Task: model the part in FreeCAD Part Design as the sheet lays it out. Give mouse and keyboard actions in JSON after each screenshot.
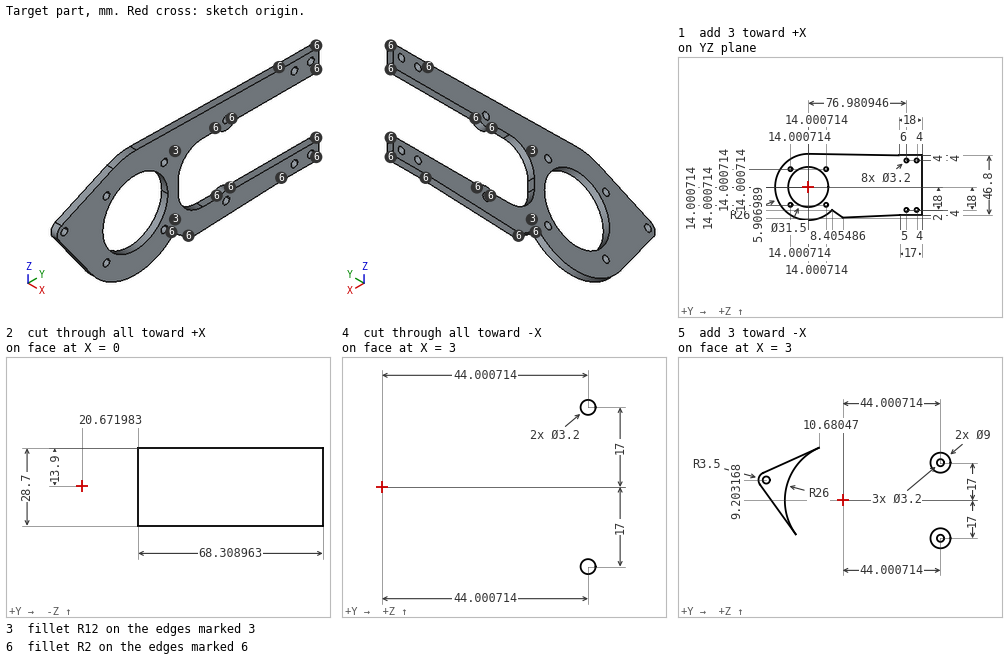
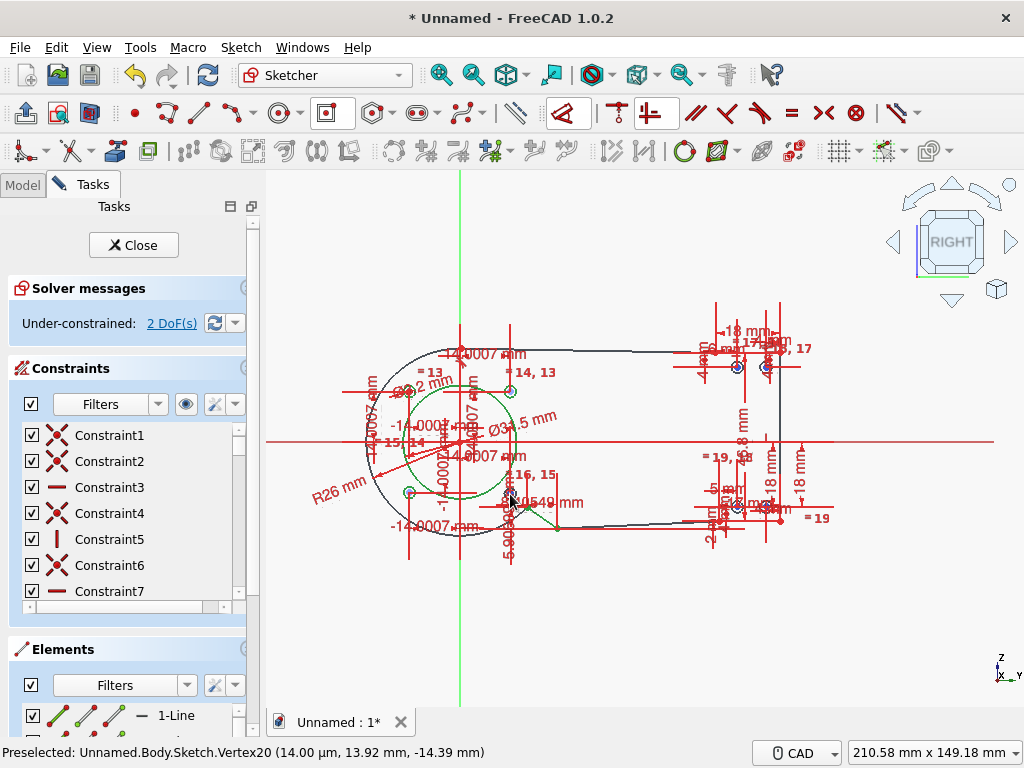
{"action": "left_click", "coordinate": [510, 494]}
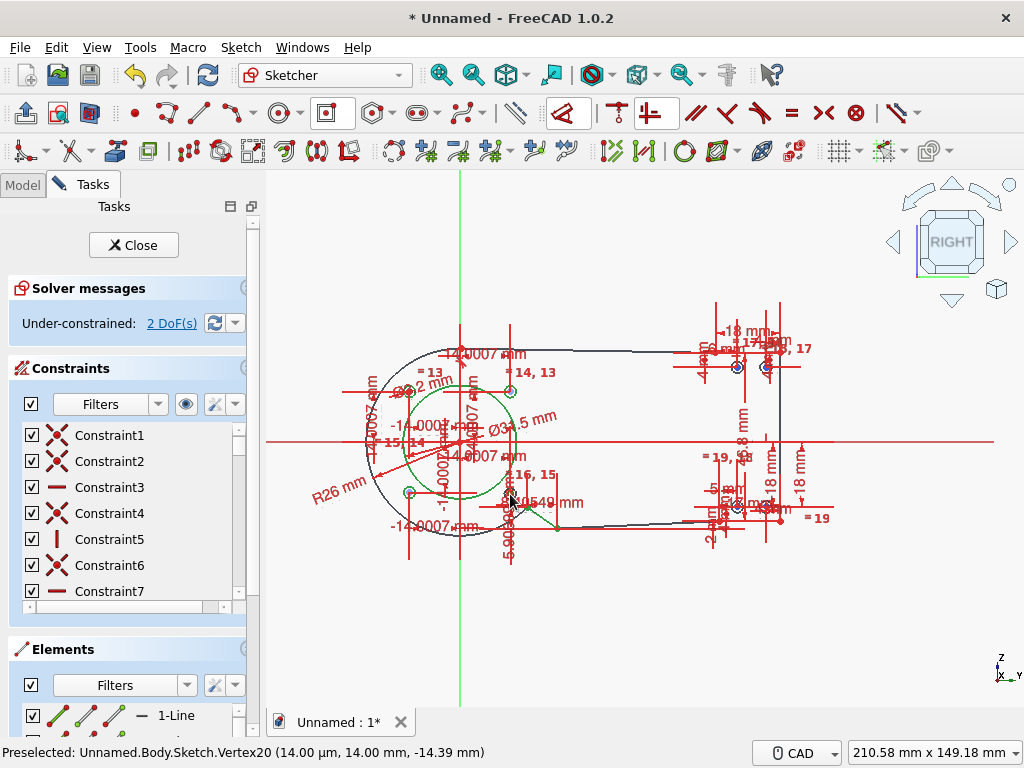
{"action": "key", "text": "i"}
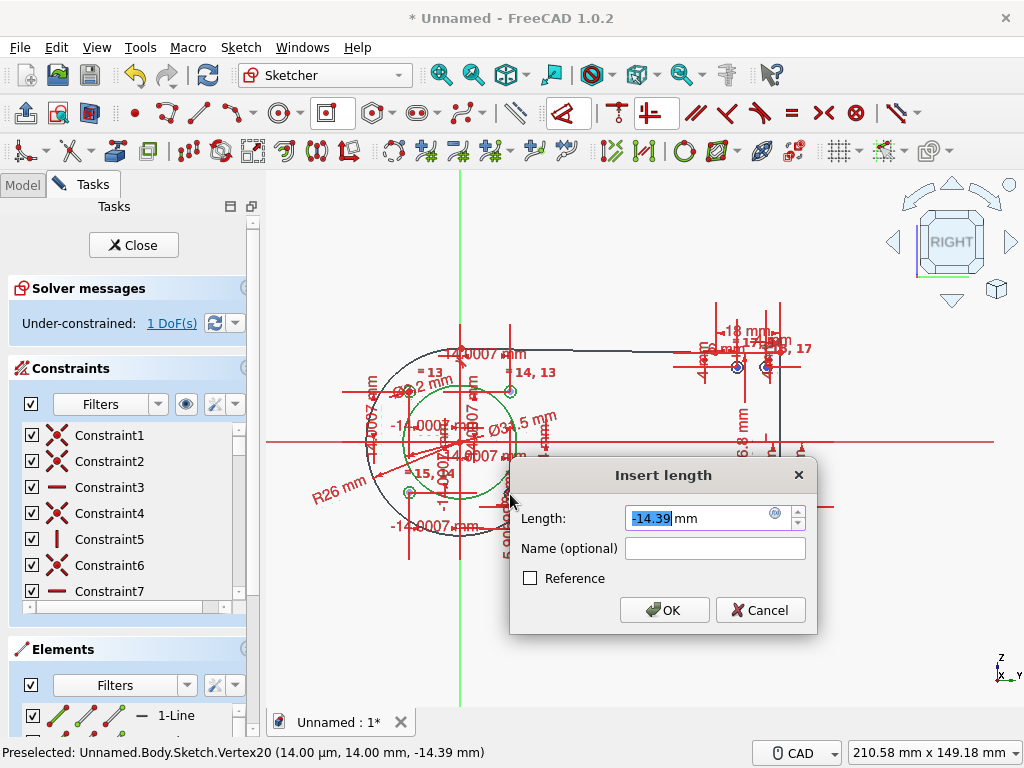
{"action": "type", "text": "-14.000714"}
{"action": "key", "text": "Return"}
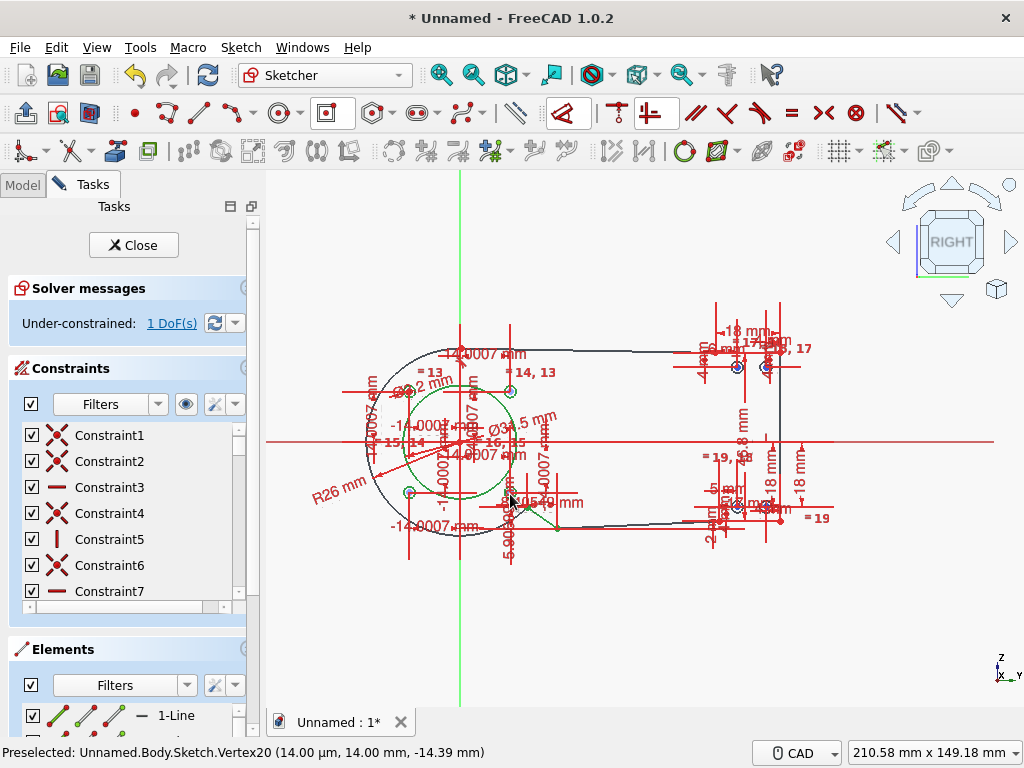
{"action": "left_click", "coordinate": [737, 367]}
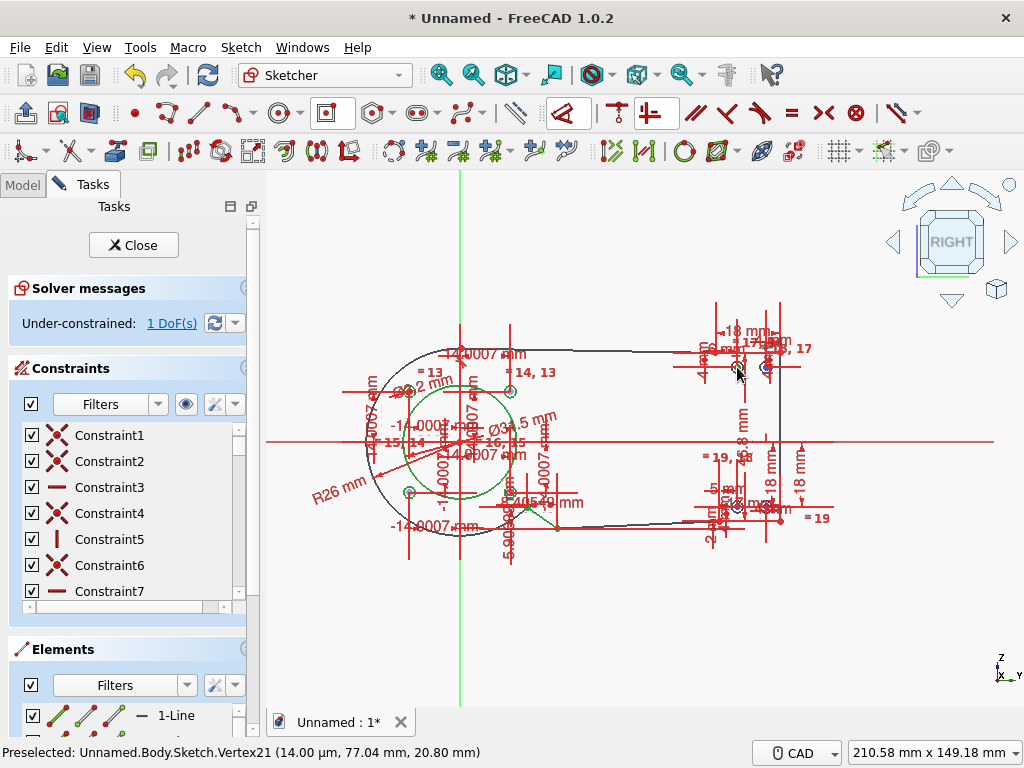
{"action": "key", "text": "l"}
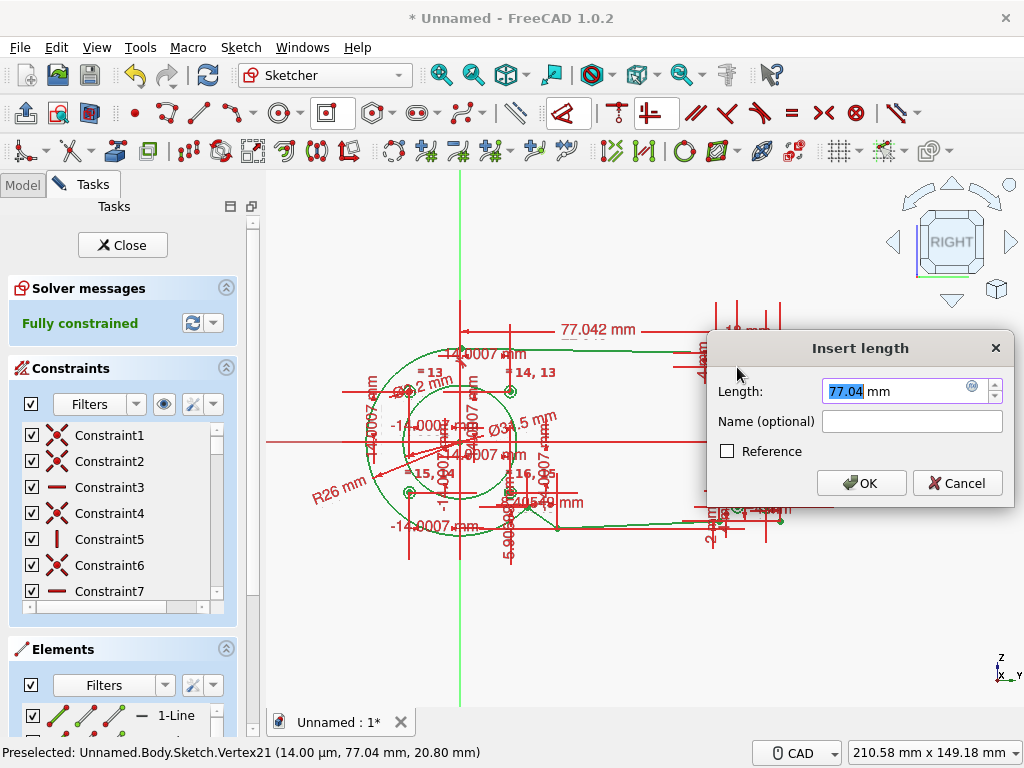
{"action": "type", "text": "76.980946"}
{"action": "key", "text": "Return"}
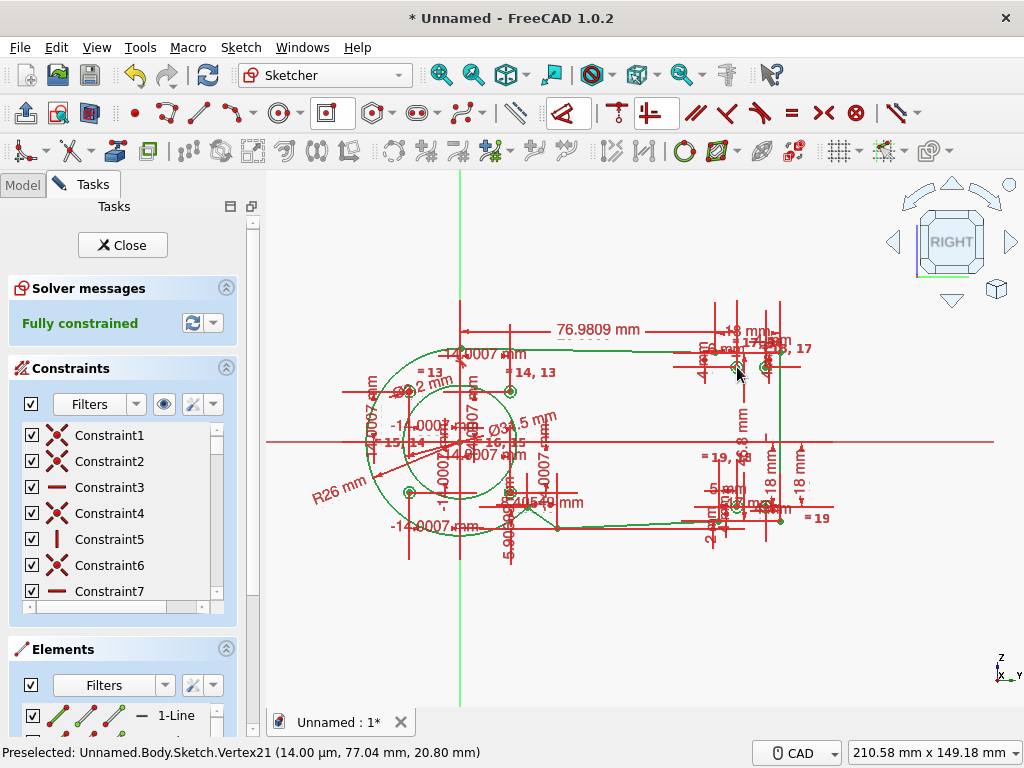
{"action": "left_click", "coordinate": [123, 245]}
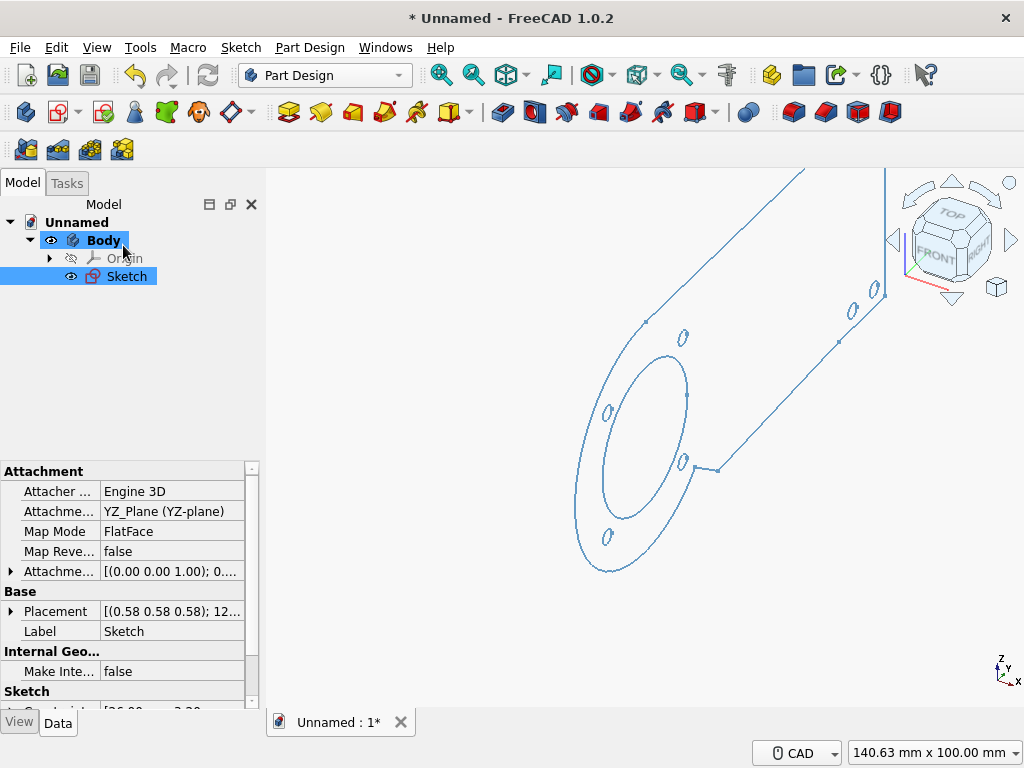
{"action": "left_click", "coordinate": [290, 112]}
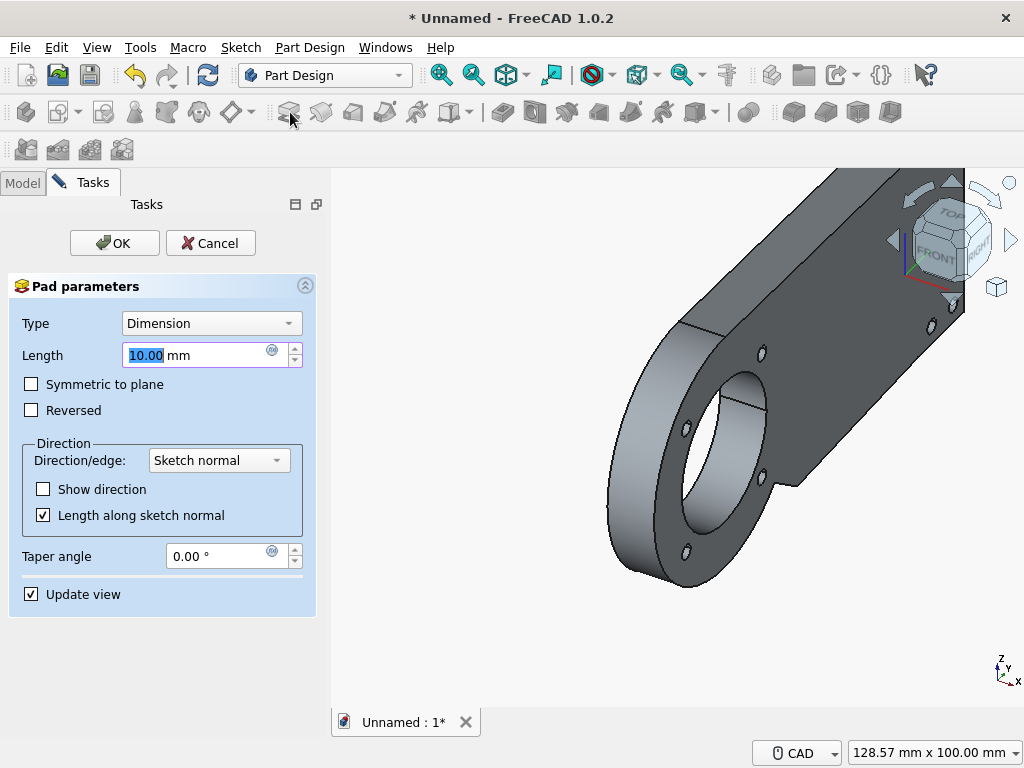
{"action": "type", "text": "3"}
{"action": "key", "text": "Tab"}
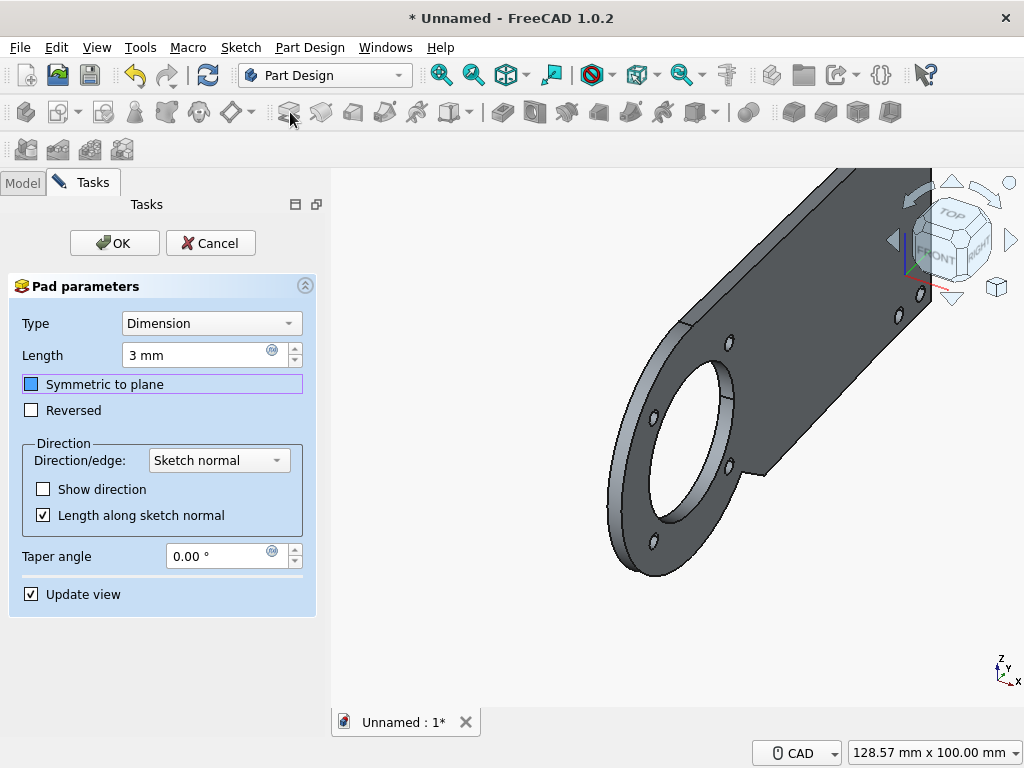
{"action": "left_click", "coordinate": [115, 243]}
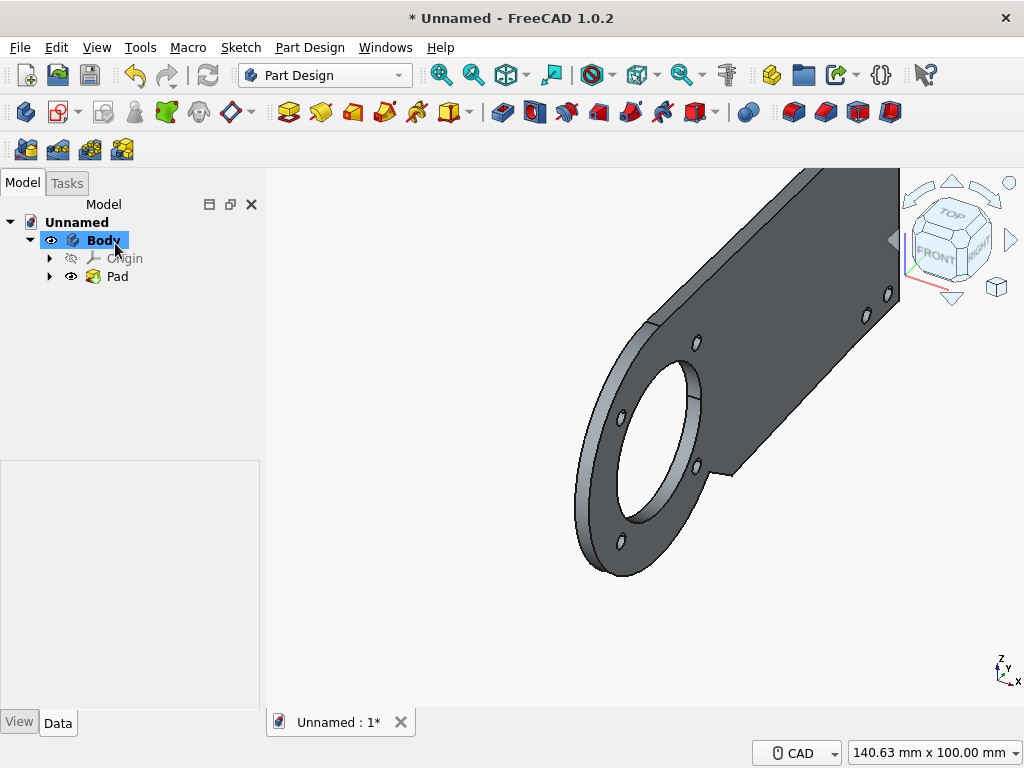
{"action": "left_click", "coordinate": [442, 76]}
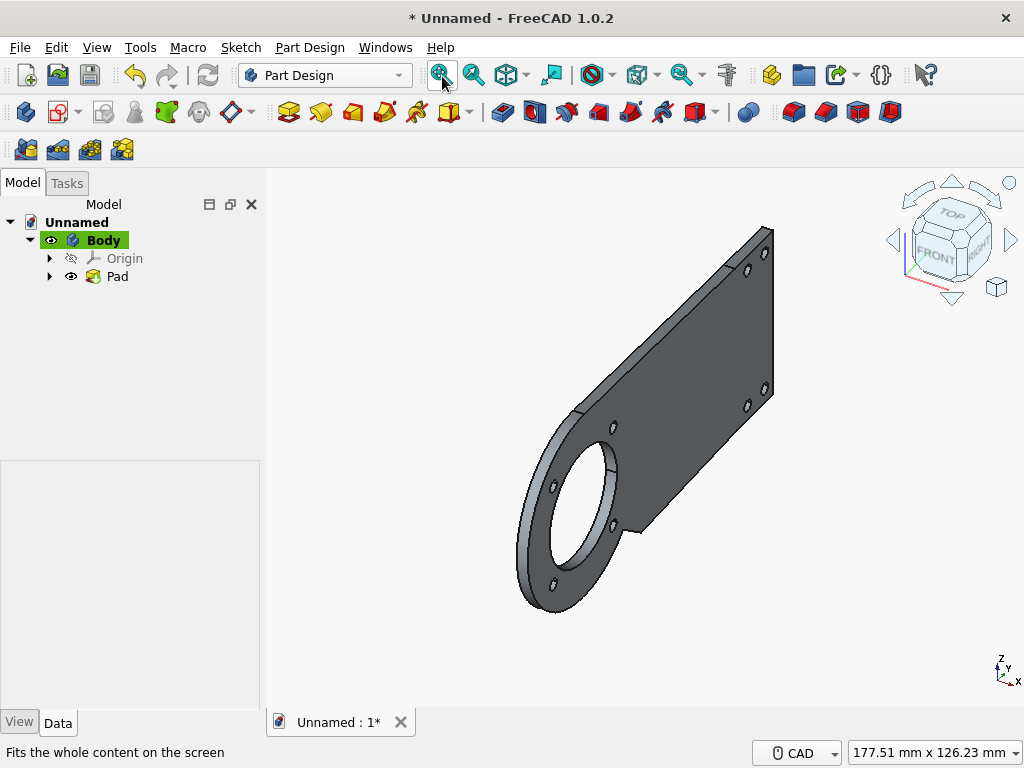
{"action": "key", "text": "6"}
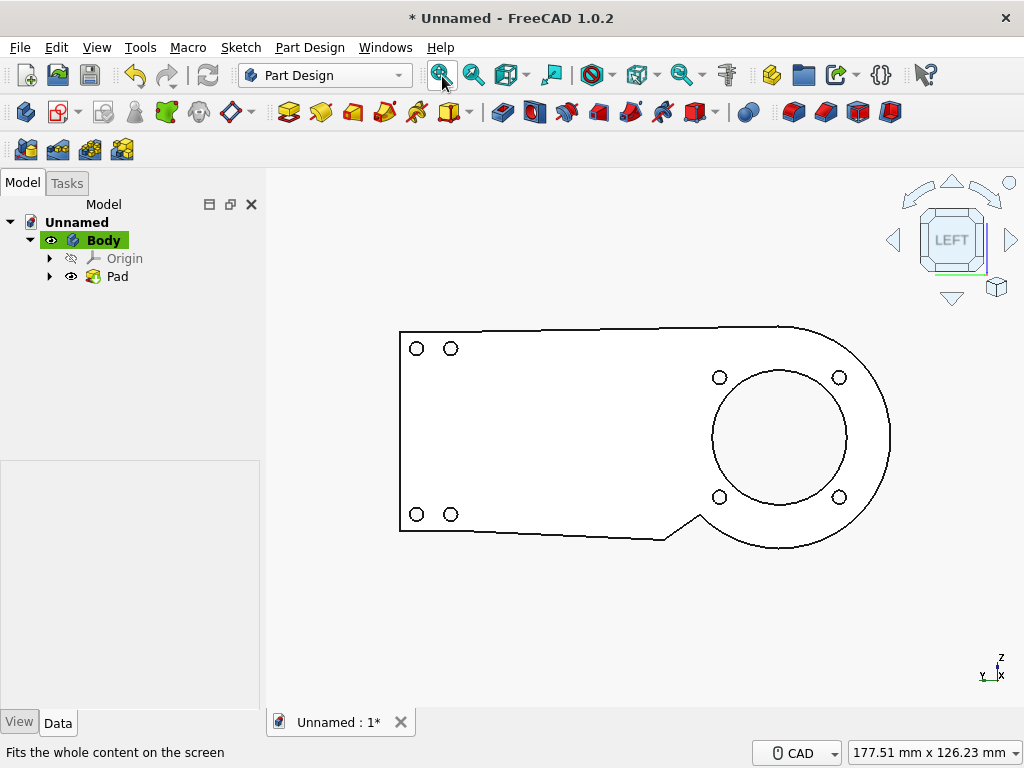
{"action": "left_click", "coordinate": [575, 436]}